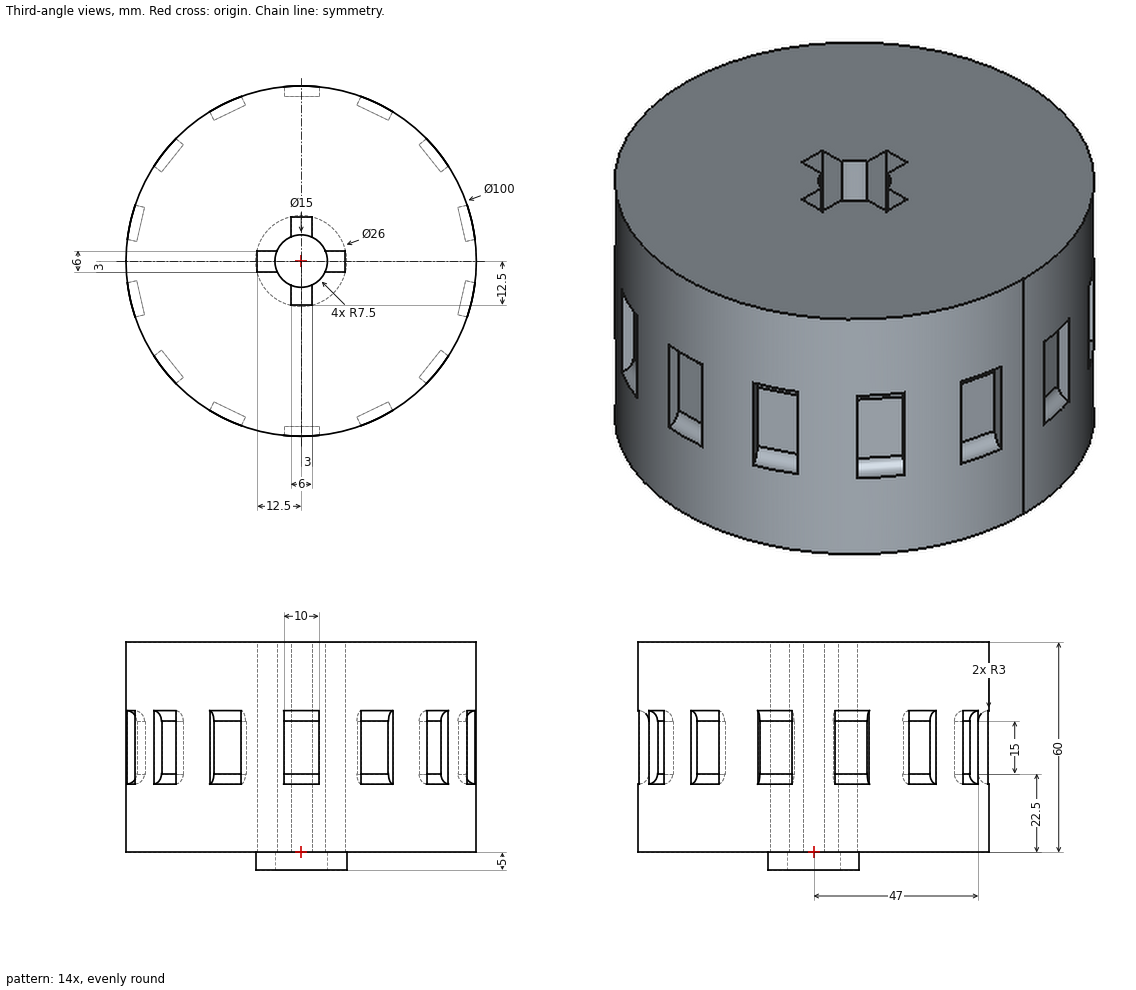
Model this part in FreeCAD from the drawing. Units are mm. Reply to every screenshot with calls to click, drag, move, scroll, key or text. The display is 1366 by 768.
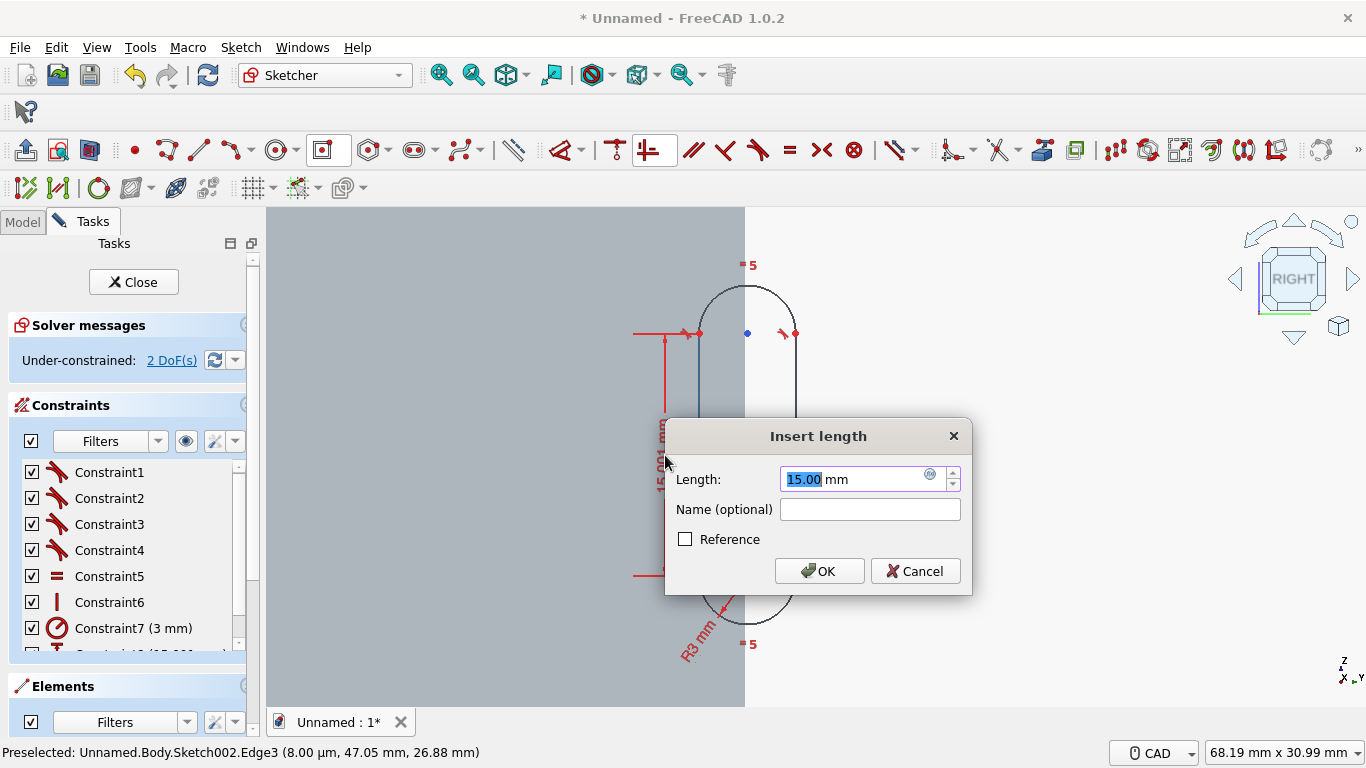
text(15)
key(Return)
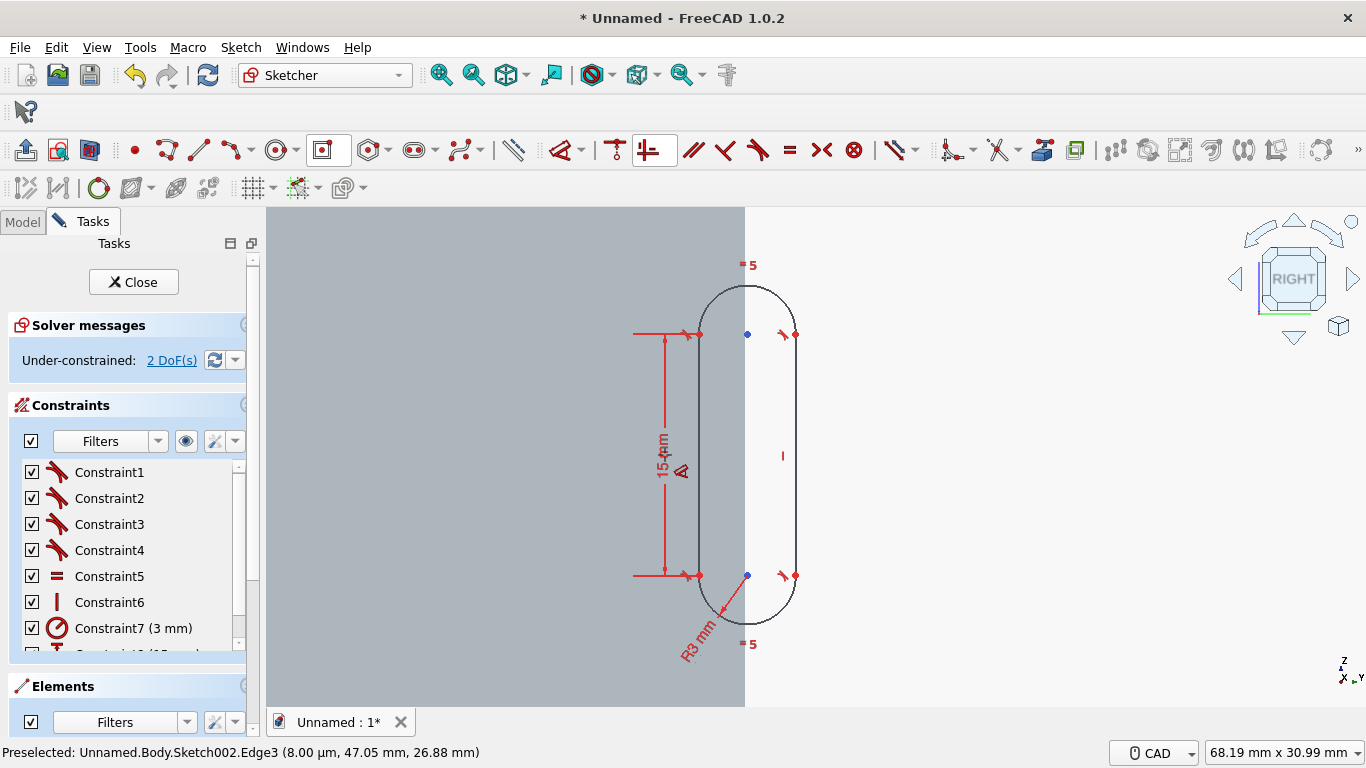
click(699, 576)
click(496, 542)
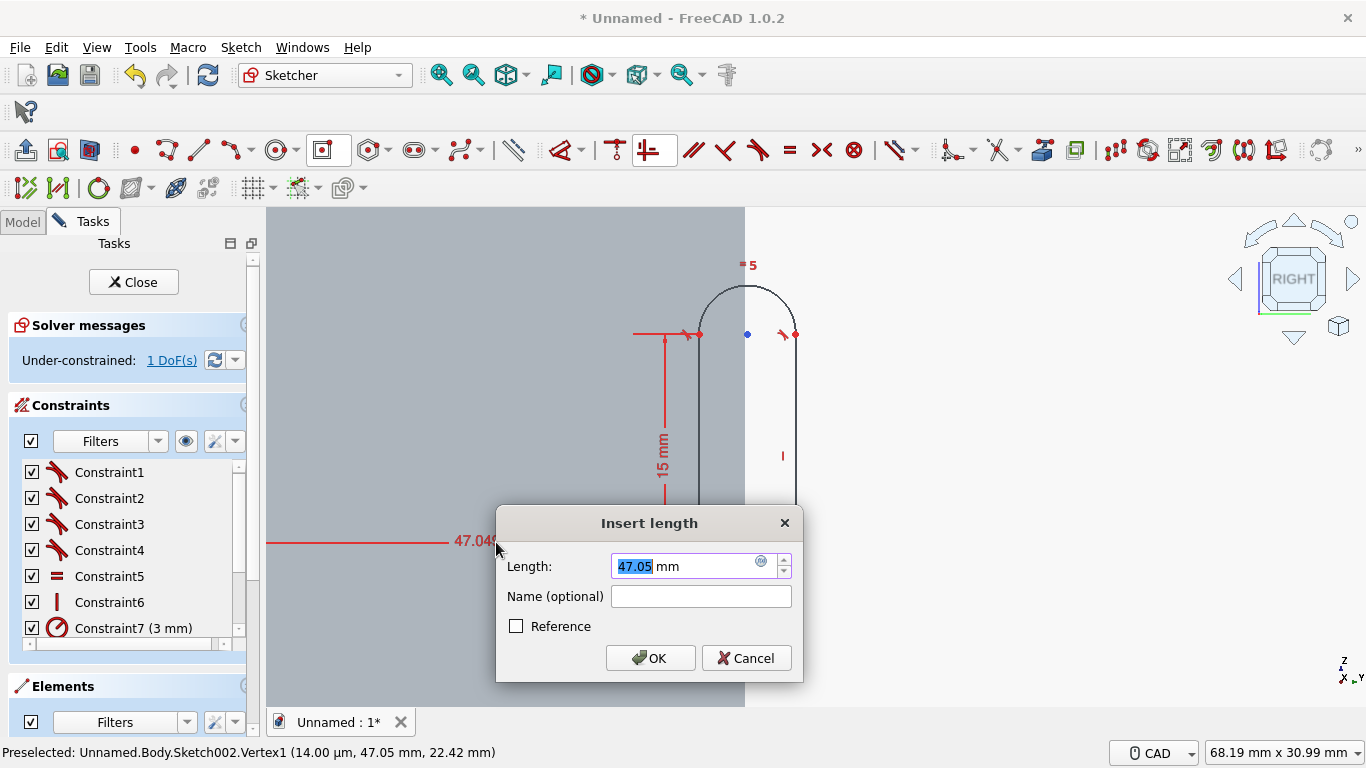
text(47)
key(Return)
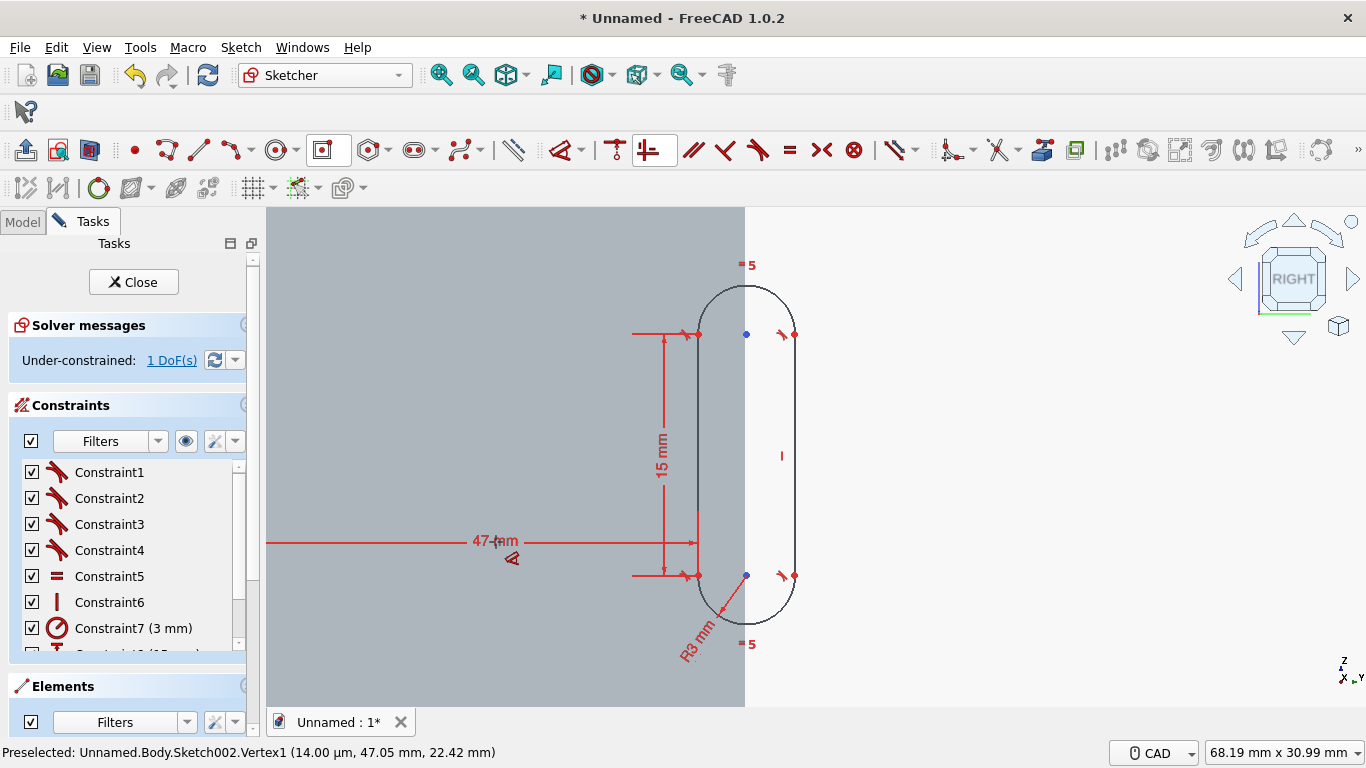
click(698, 576)
click(732, 604)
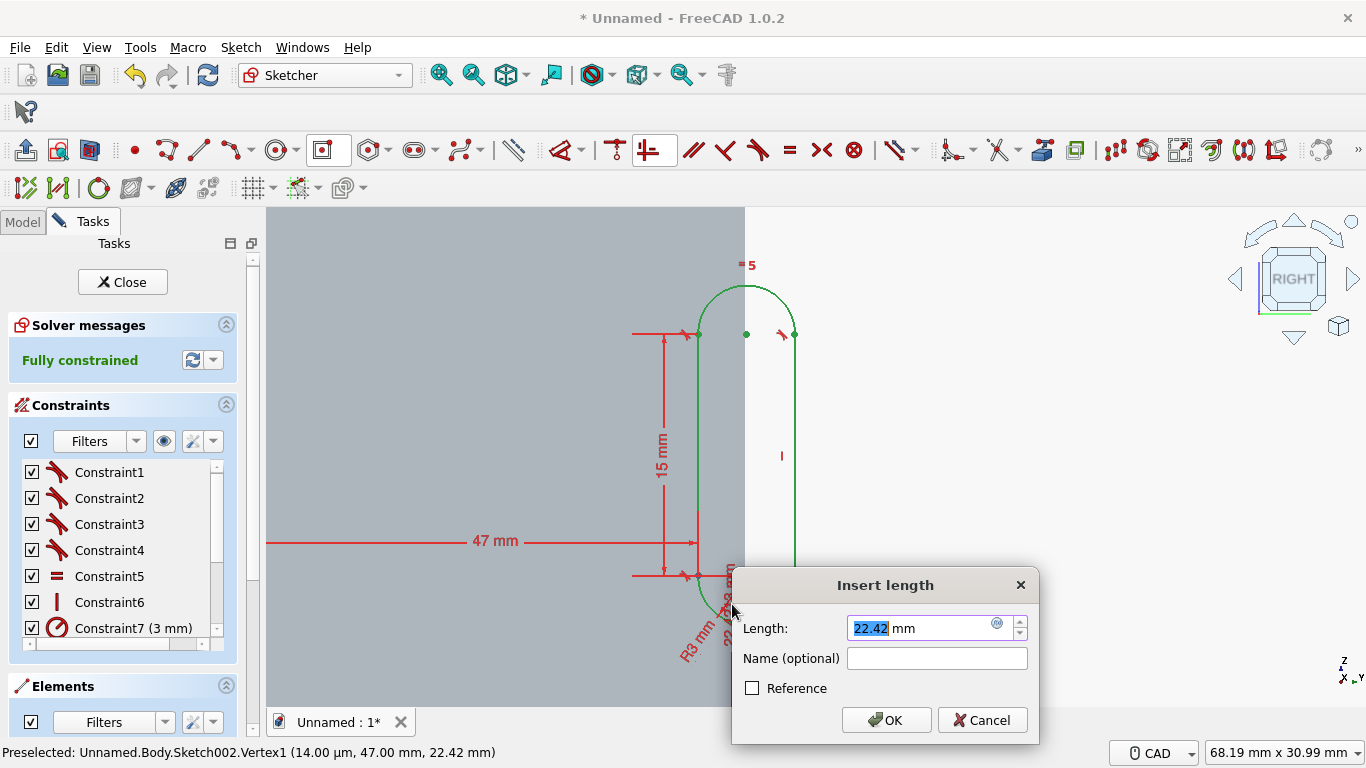
text(22.5)
key(Return)
key(Escape)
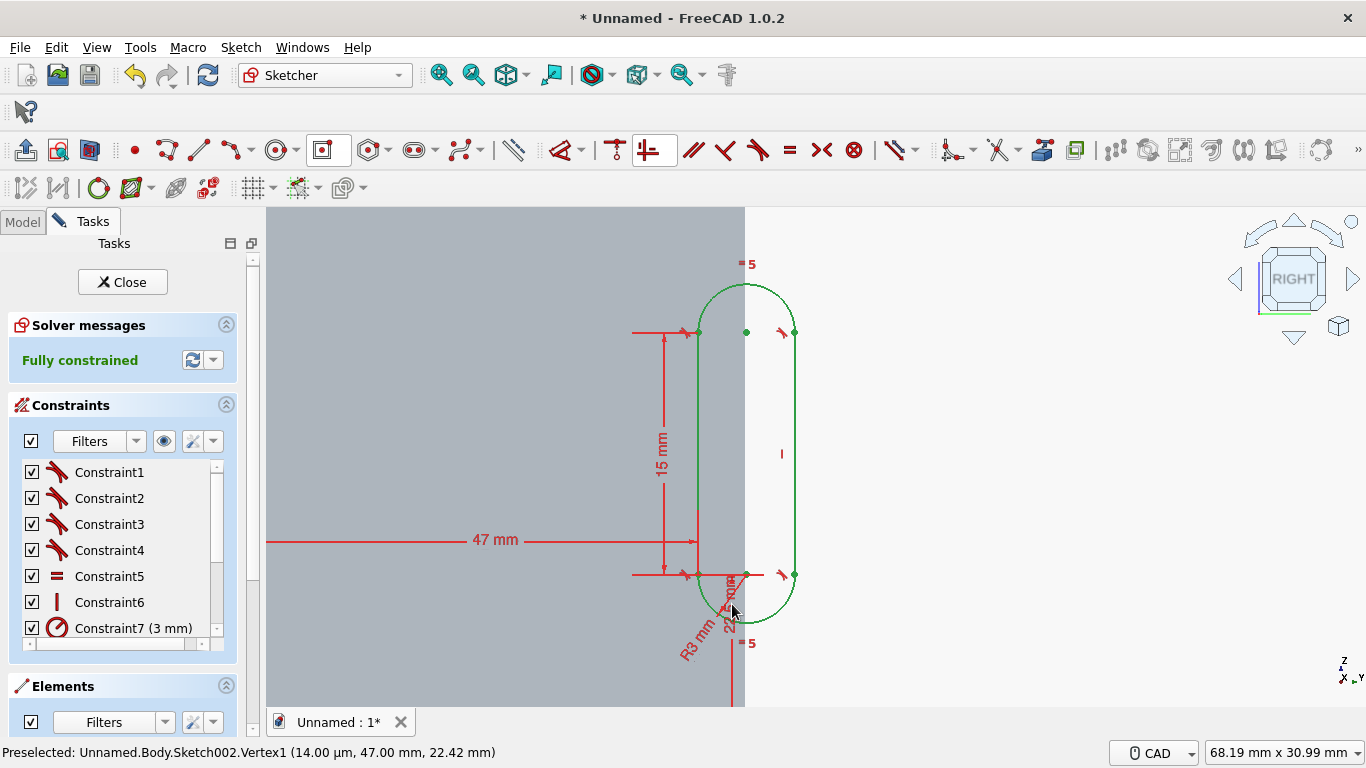
click(123, 282)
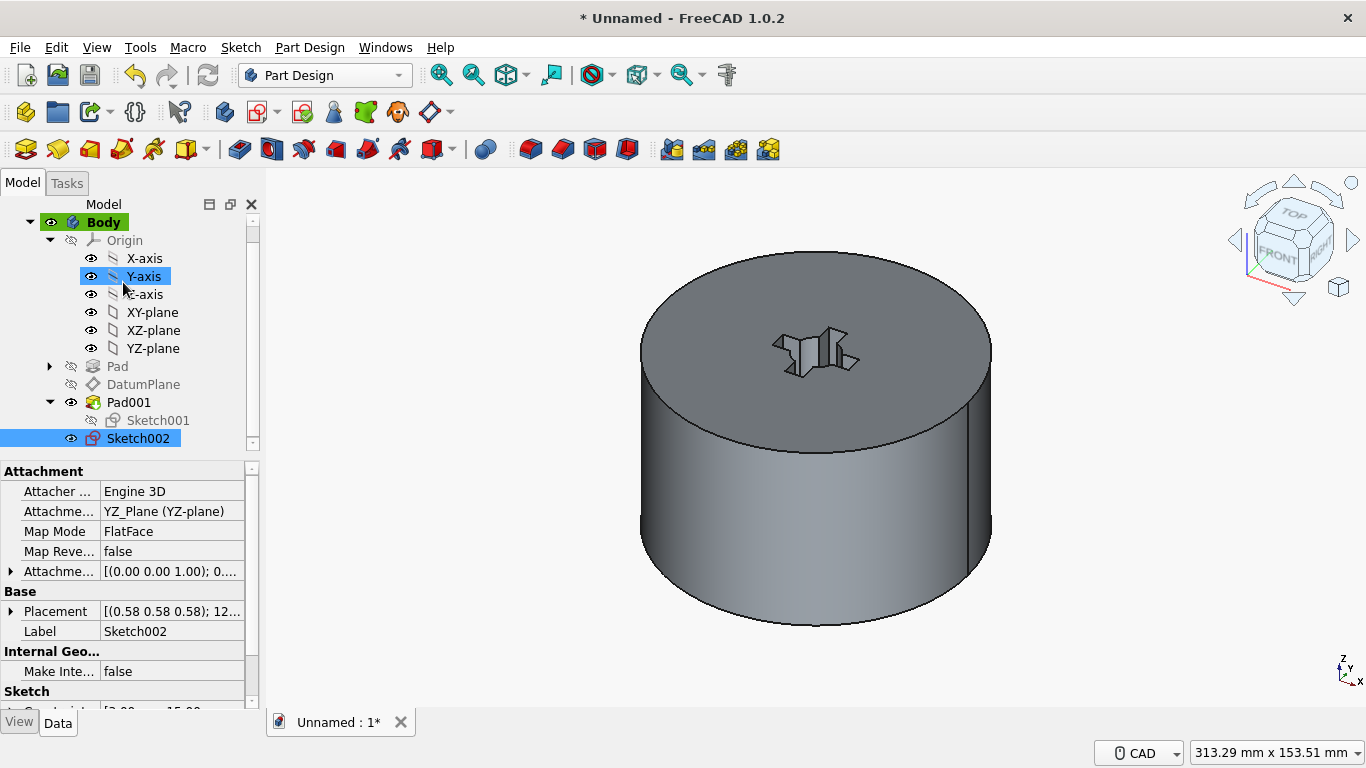
click(240, 150)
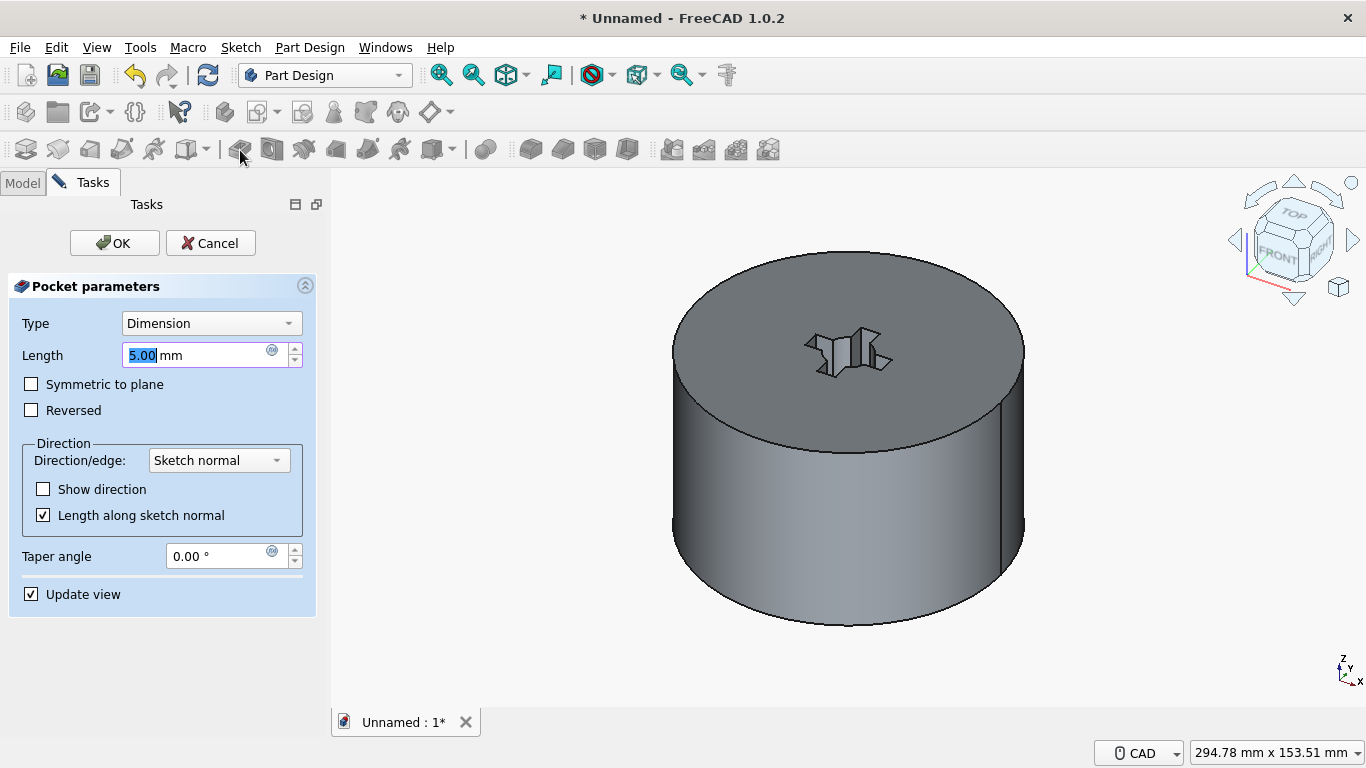
text(10)
key(Tab)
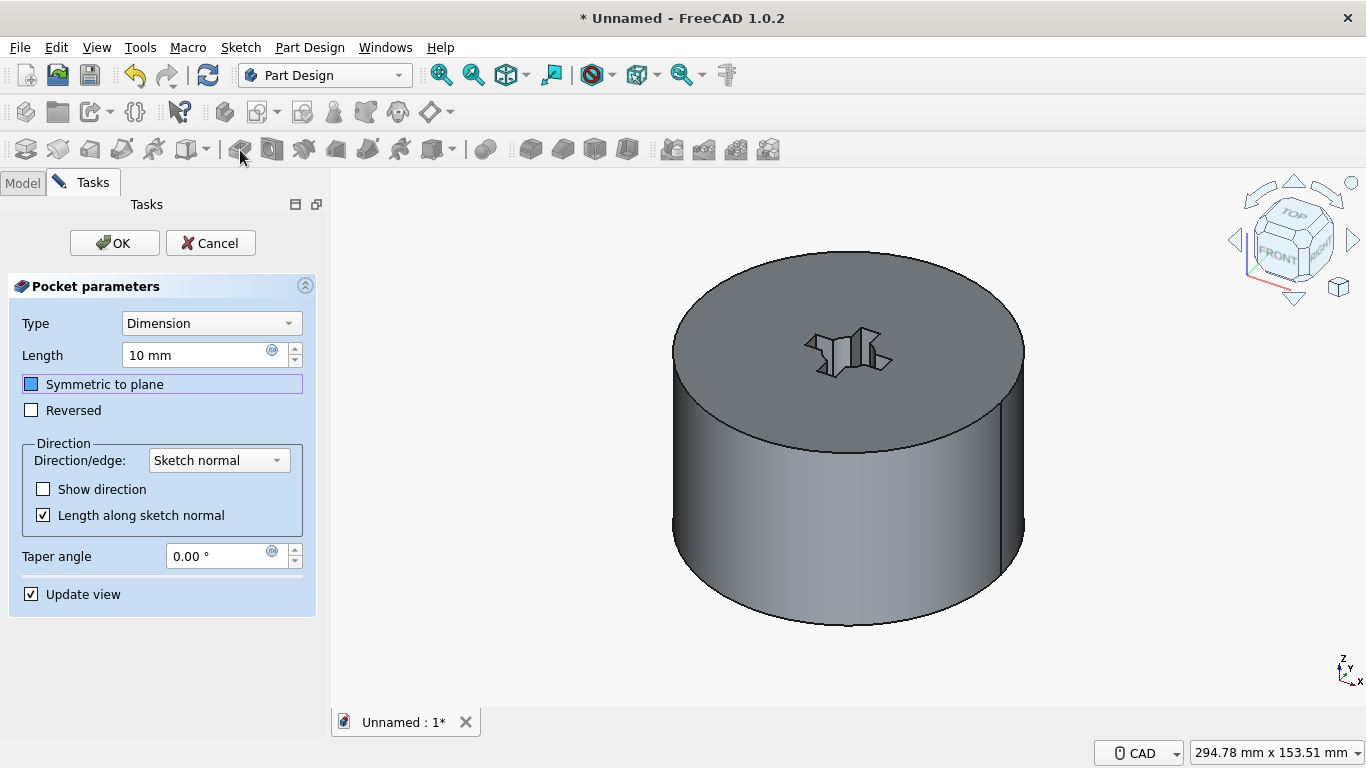
click(30, 384)